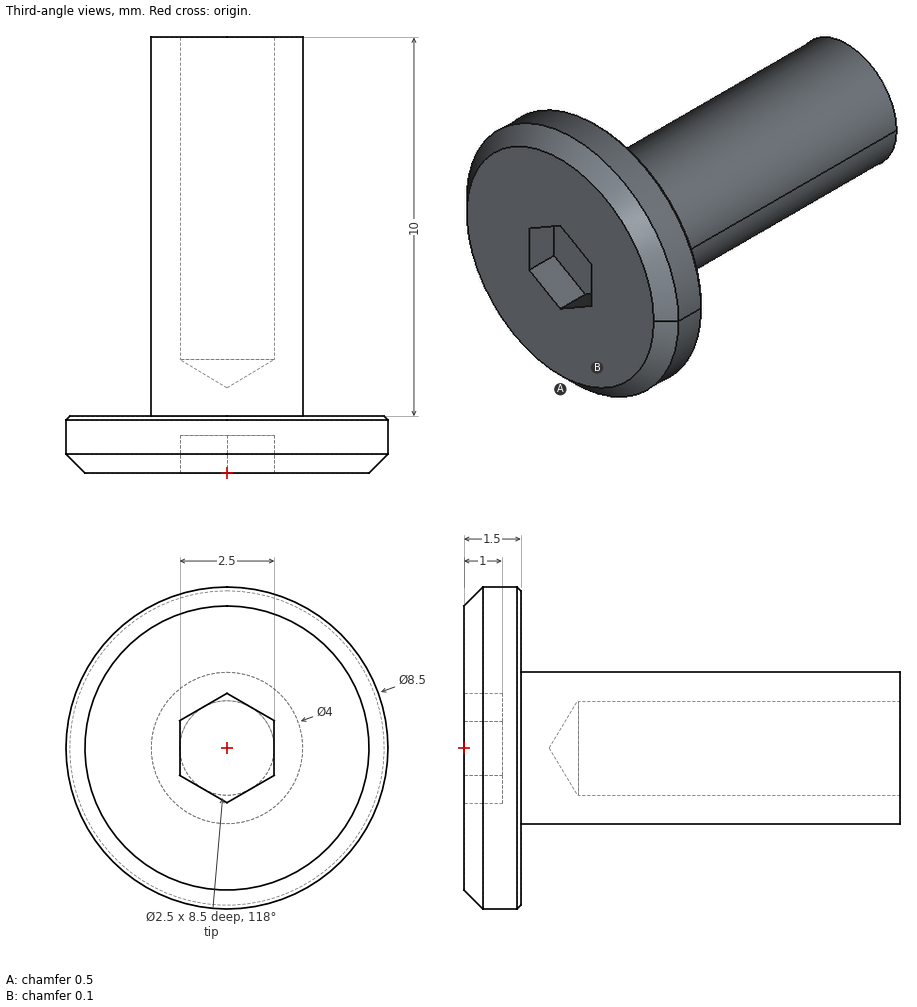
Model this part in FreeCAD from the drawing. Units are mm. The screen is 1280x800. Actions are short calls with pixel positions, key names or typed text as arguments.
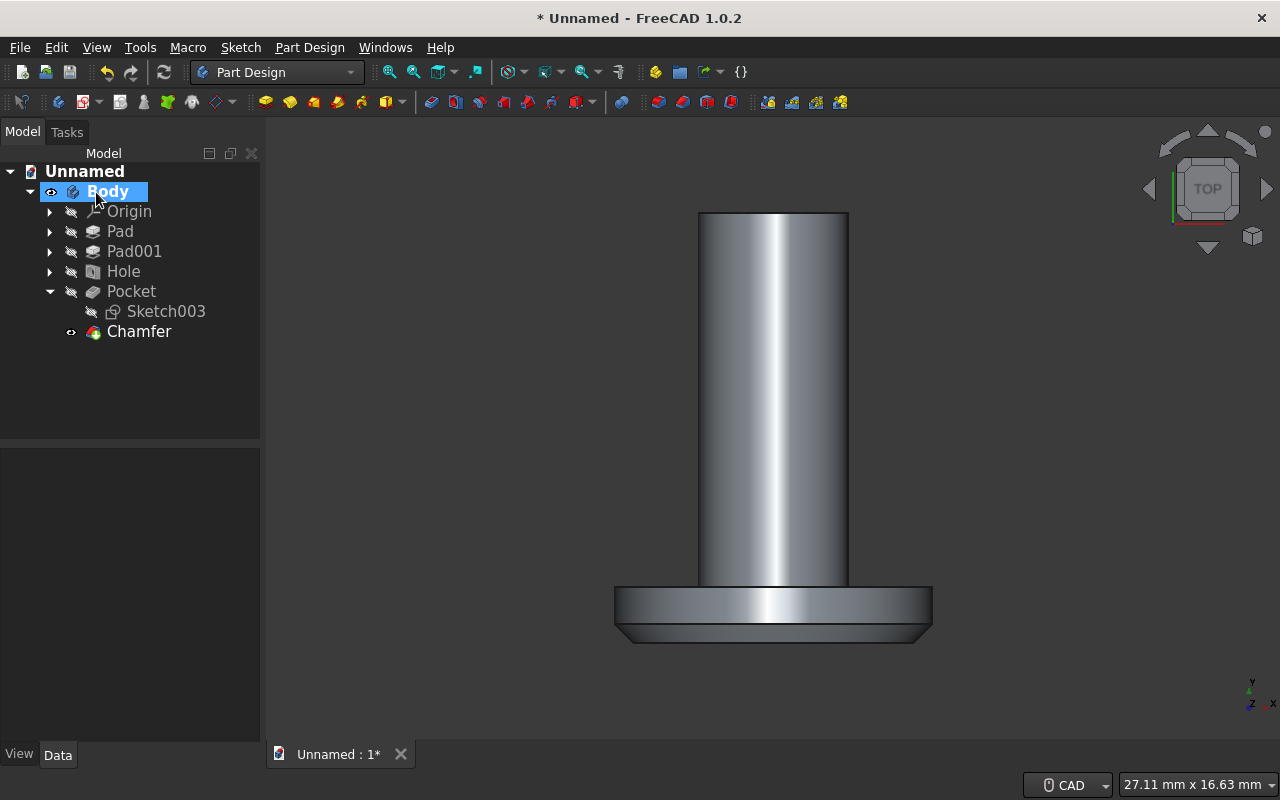
click(644, 586)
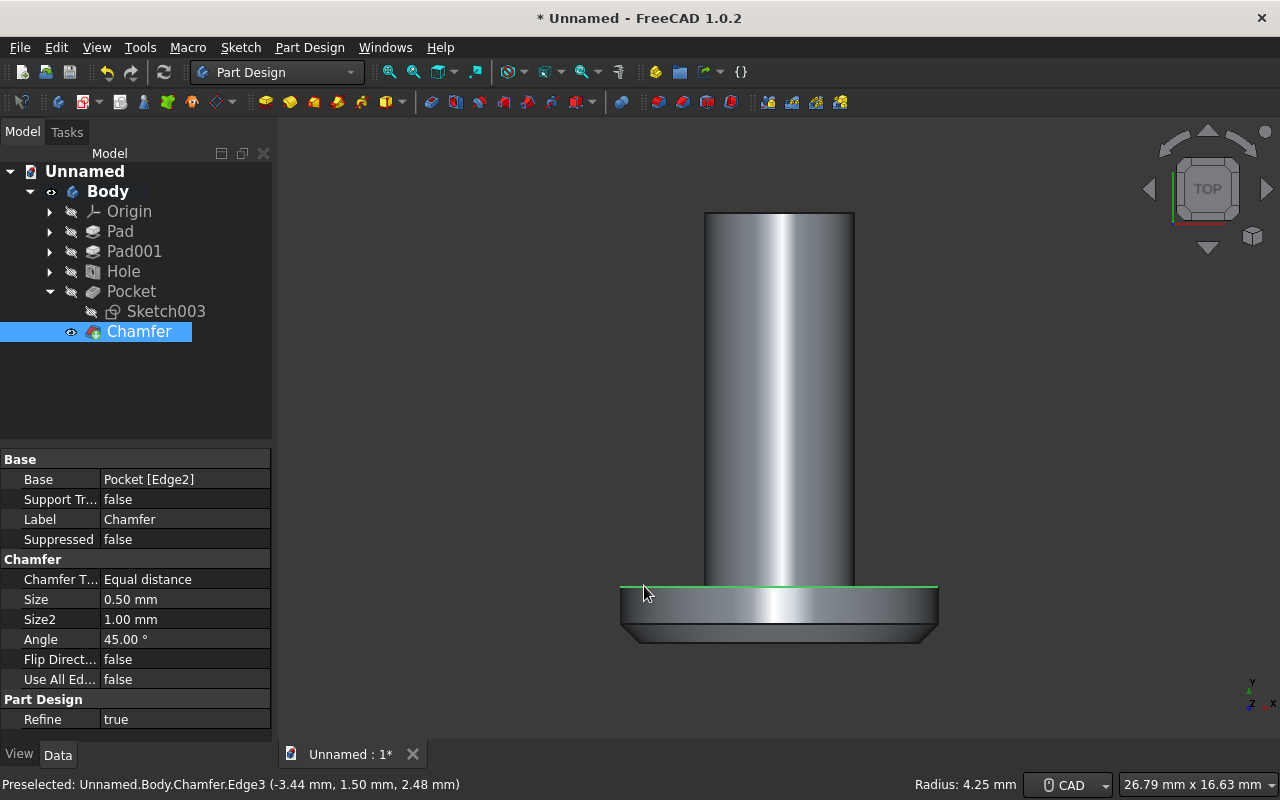
click(684, 102)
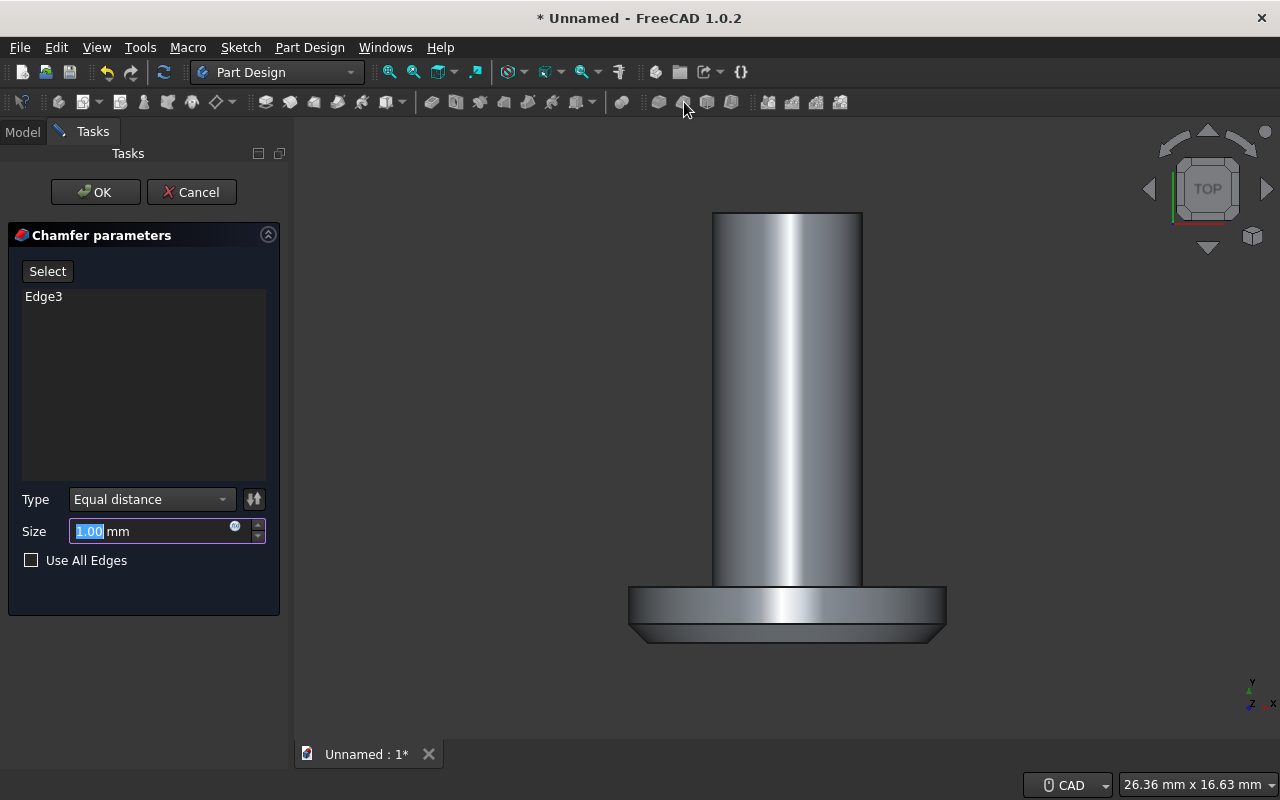
text(0.1)
key(Tab)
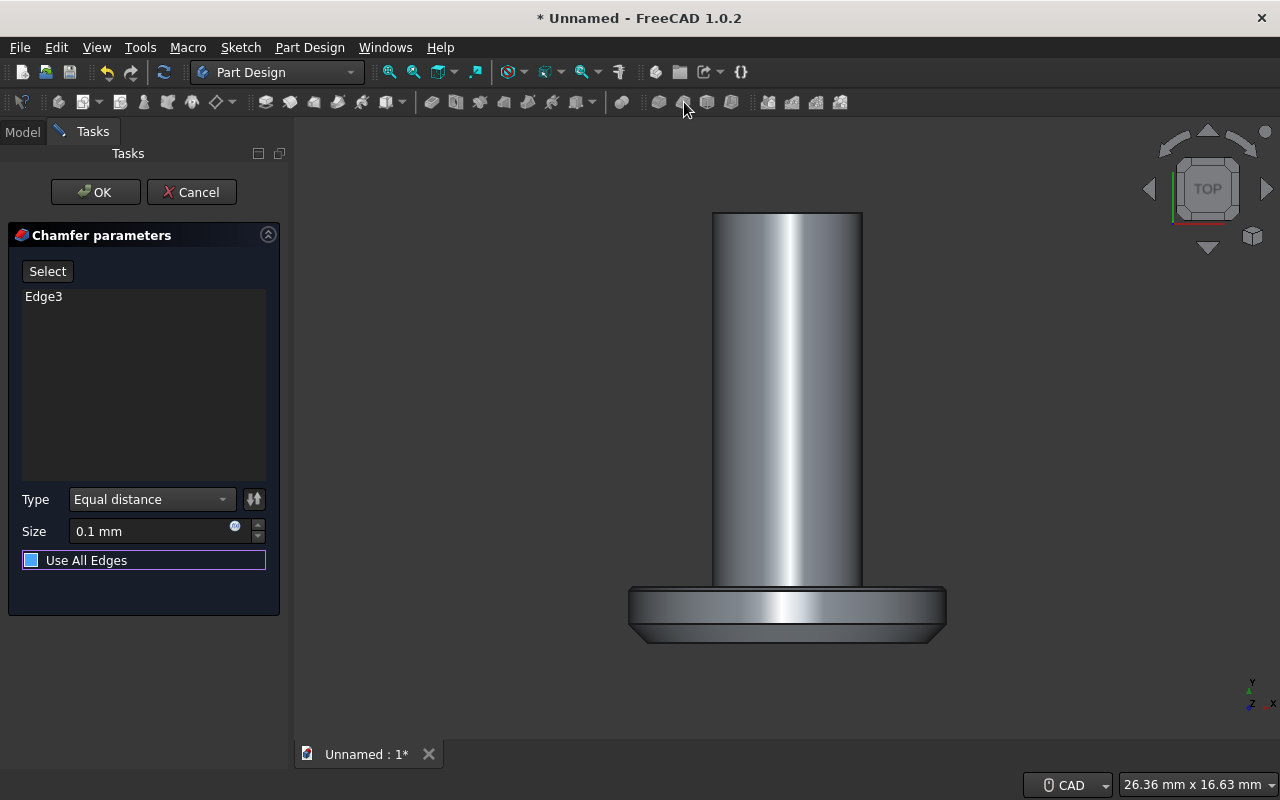
click(96, 192)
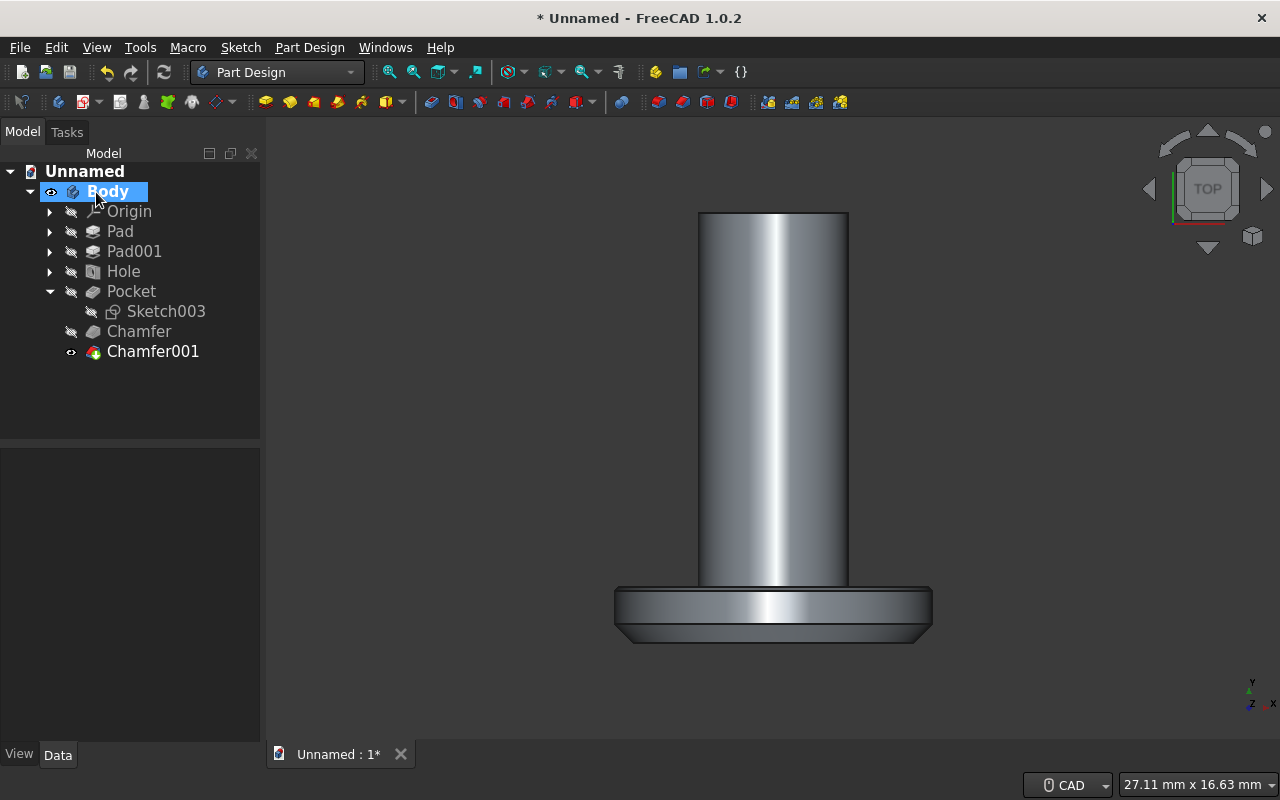
key(0)